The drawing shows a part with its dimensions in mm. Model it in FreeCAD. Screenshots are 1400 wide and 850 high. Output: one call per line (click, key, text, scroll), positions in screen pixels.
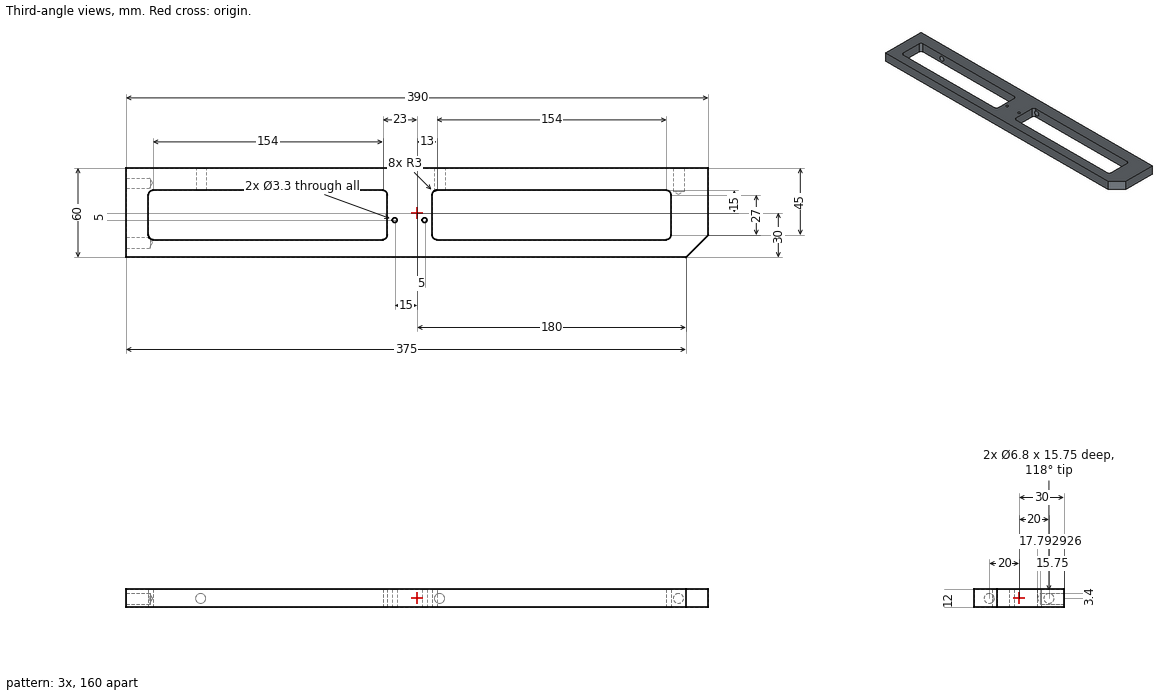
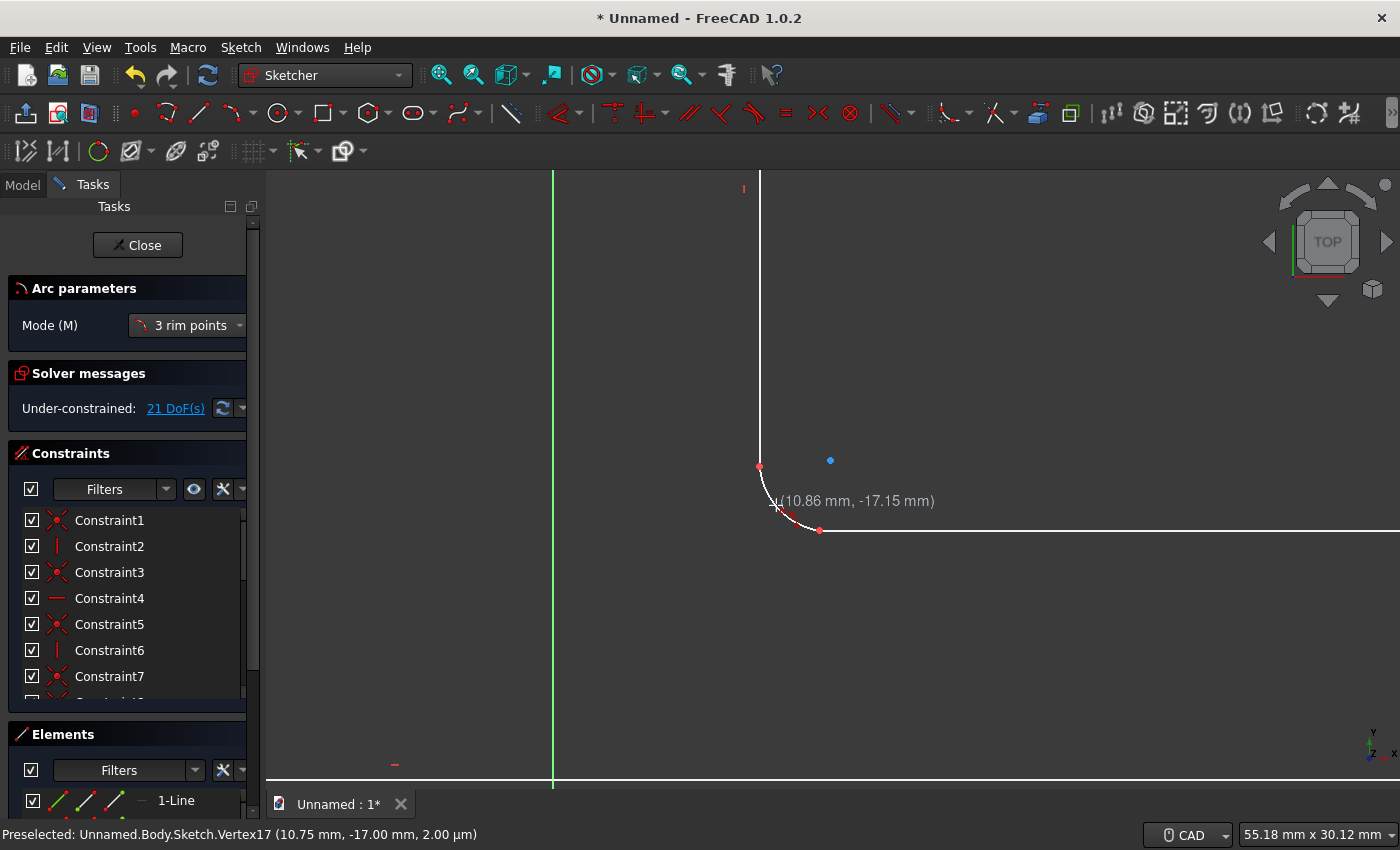
scroll(786, 512, down, 12)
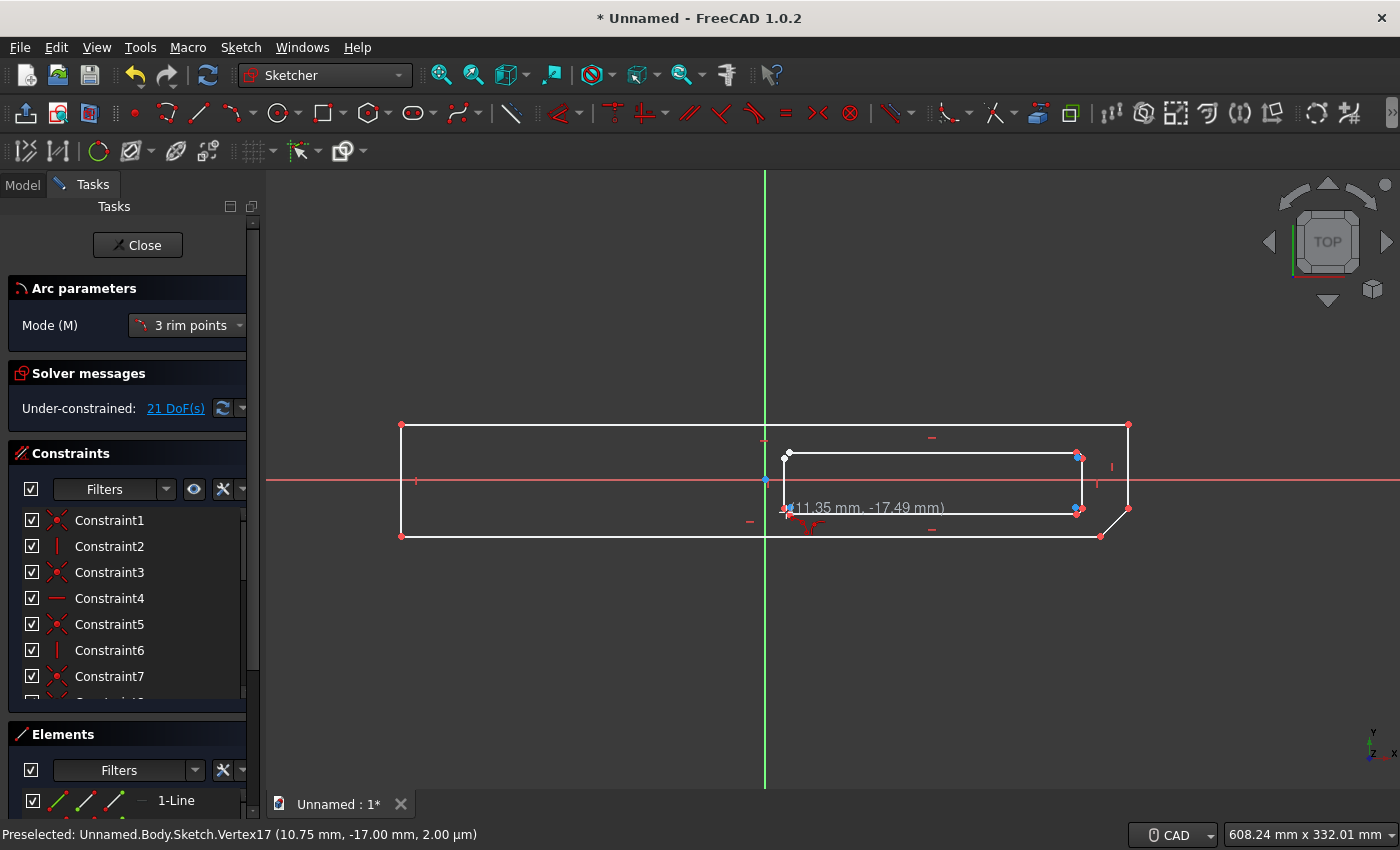
scroll(784, 458, up, 4)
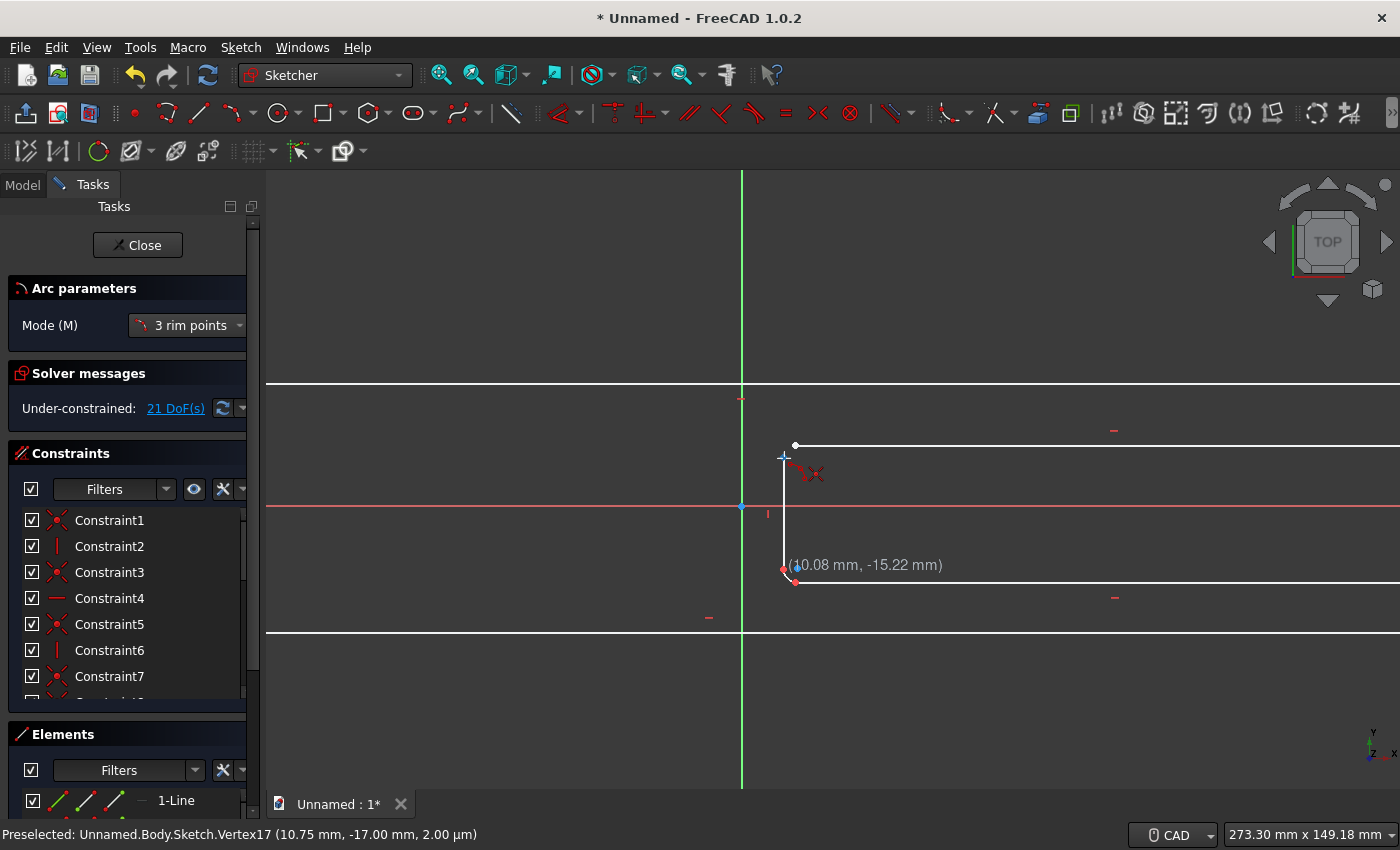
click(784, 458)
click(796, 446)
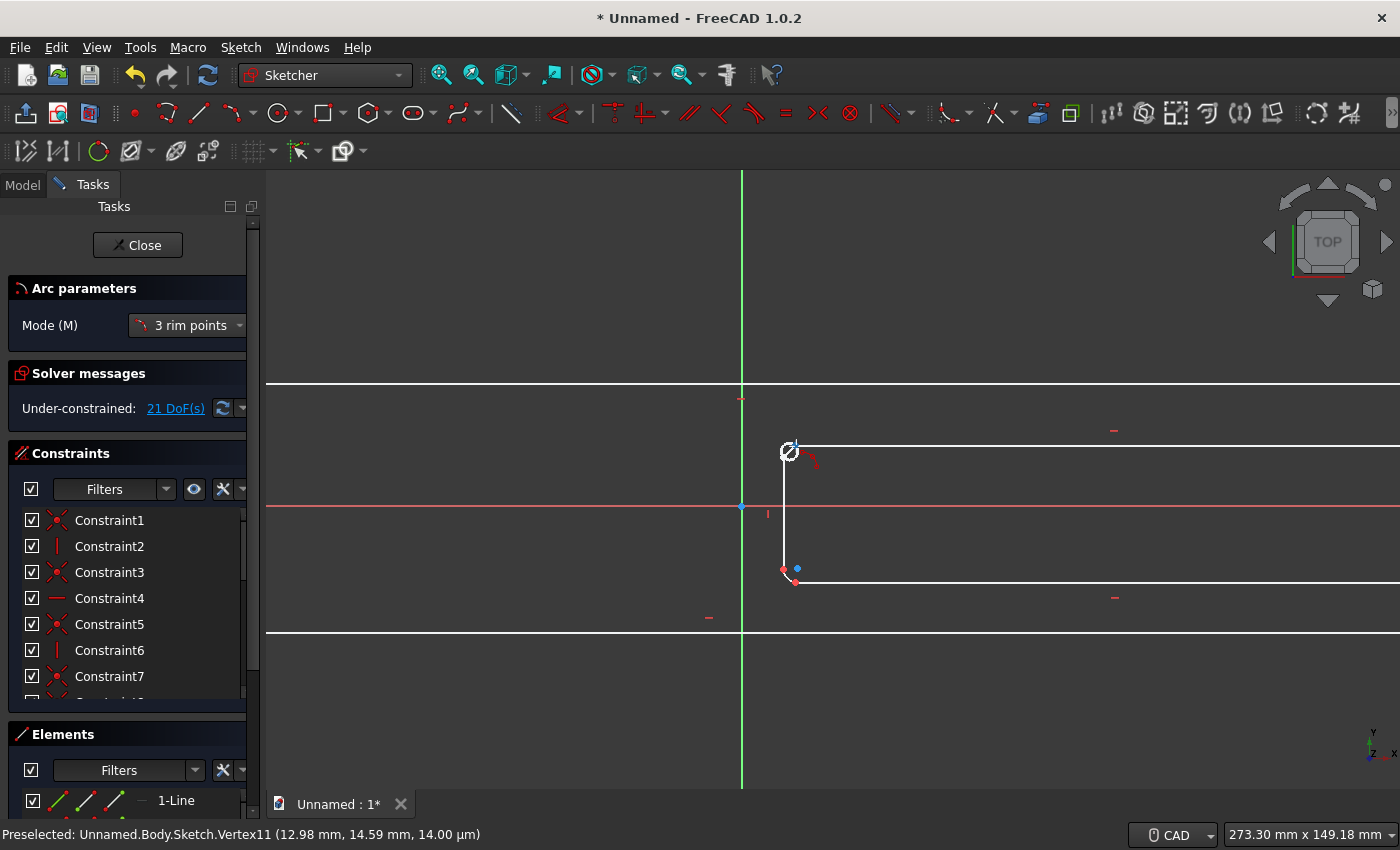
scroll(787, 448, up, 8)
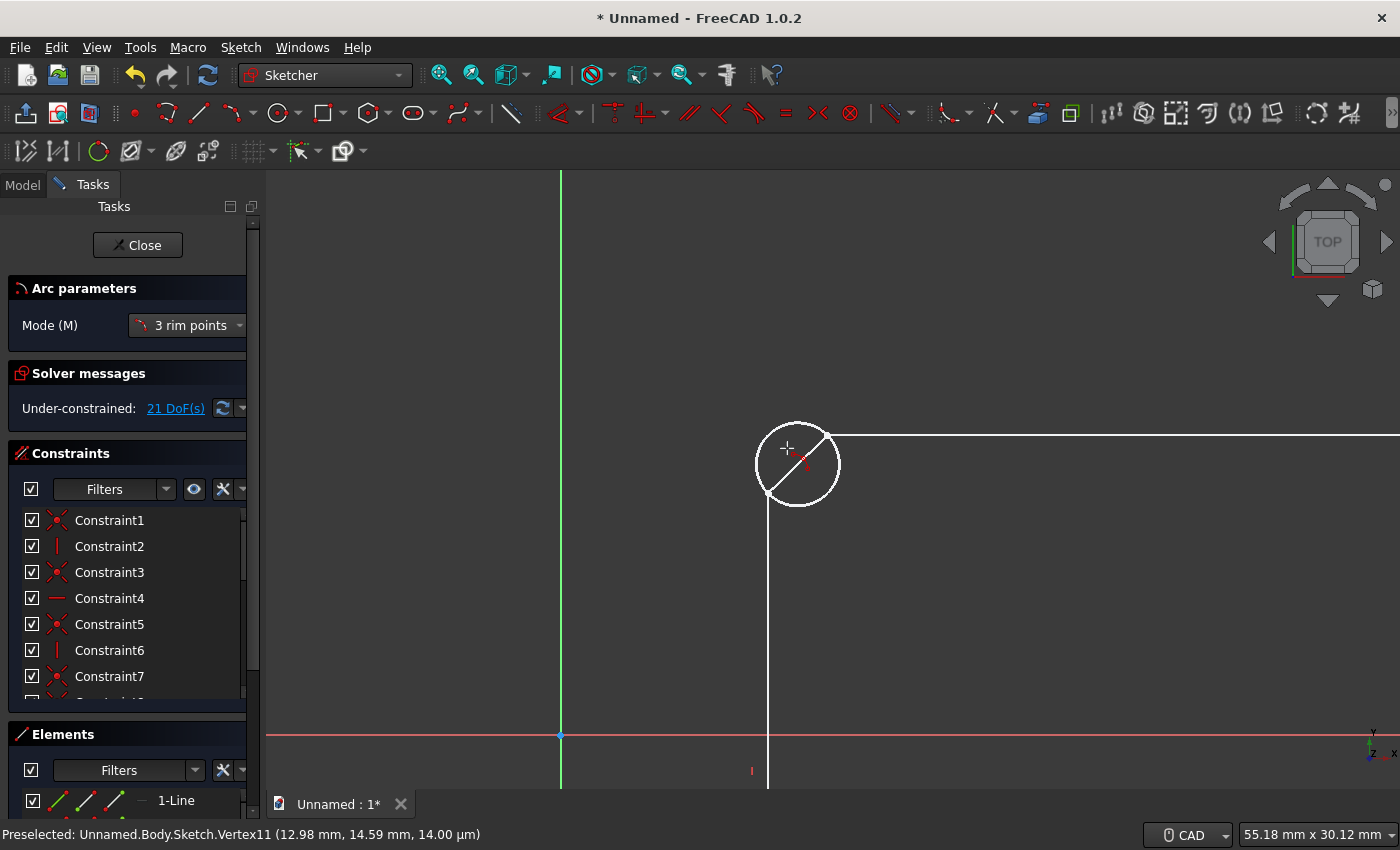
click(784, 445)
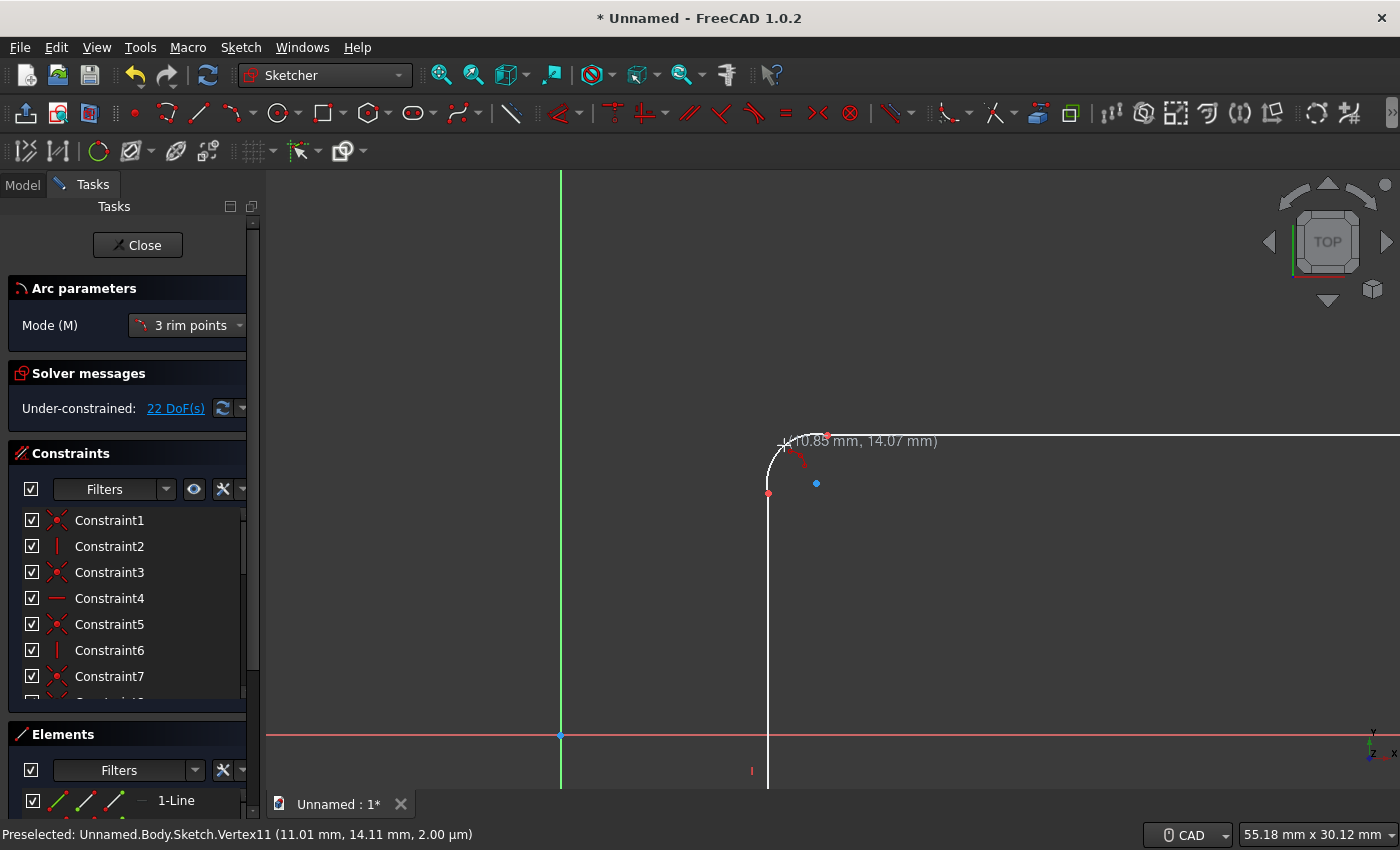
click(200, 114)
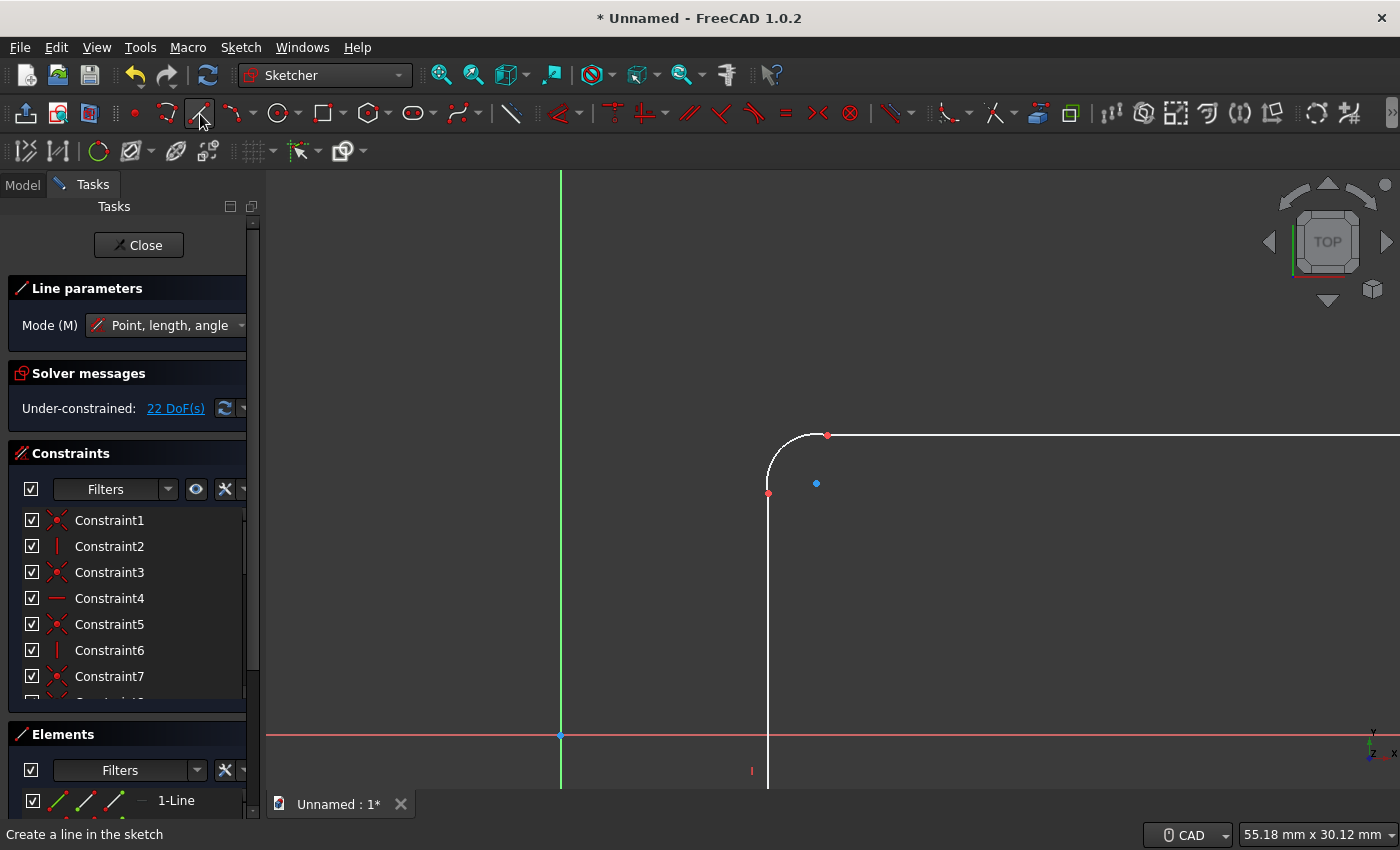
scroll(785, 454, down, 12)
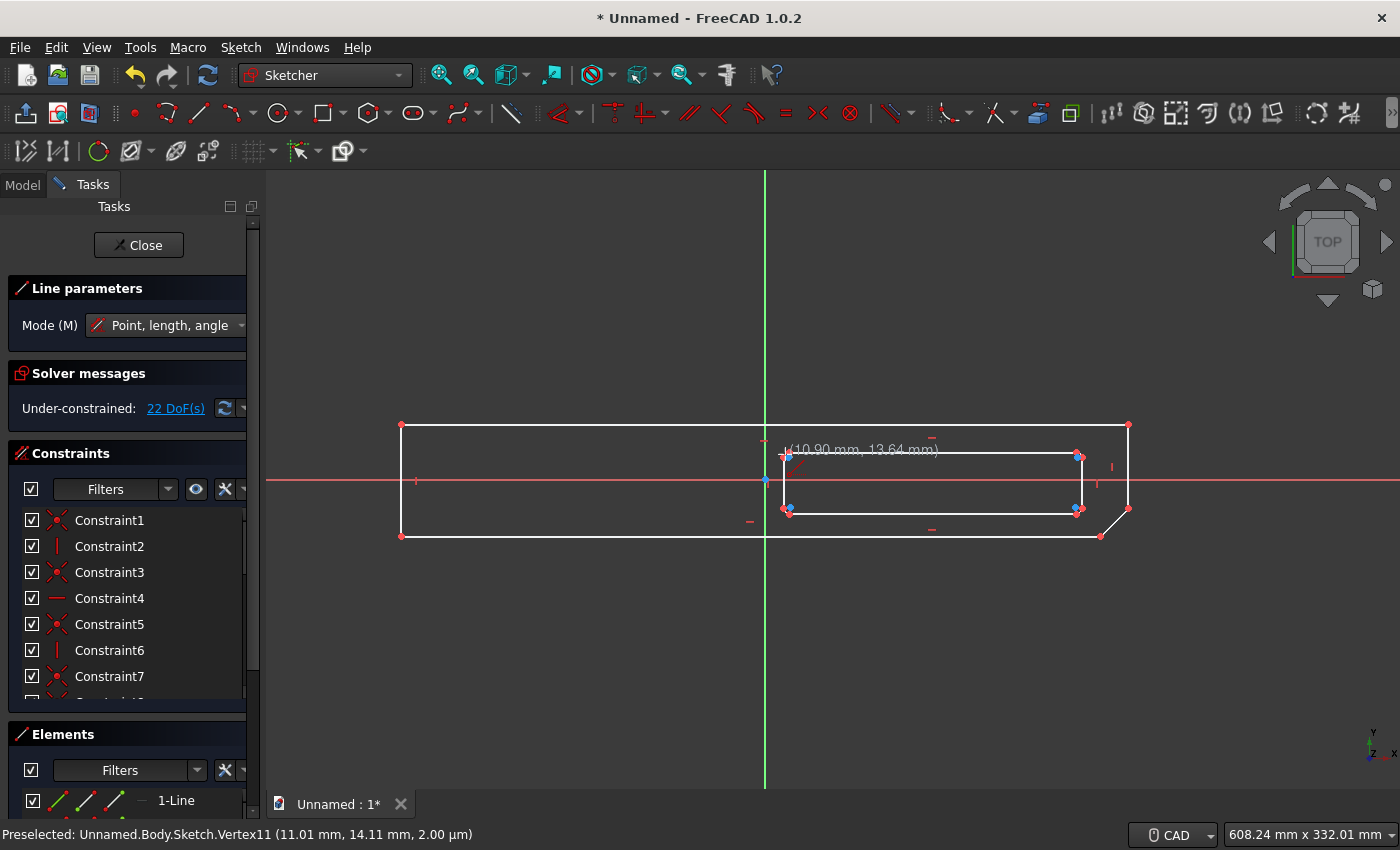
click(435, 452)
click(722, 452)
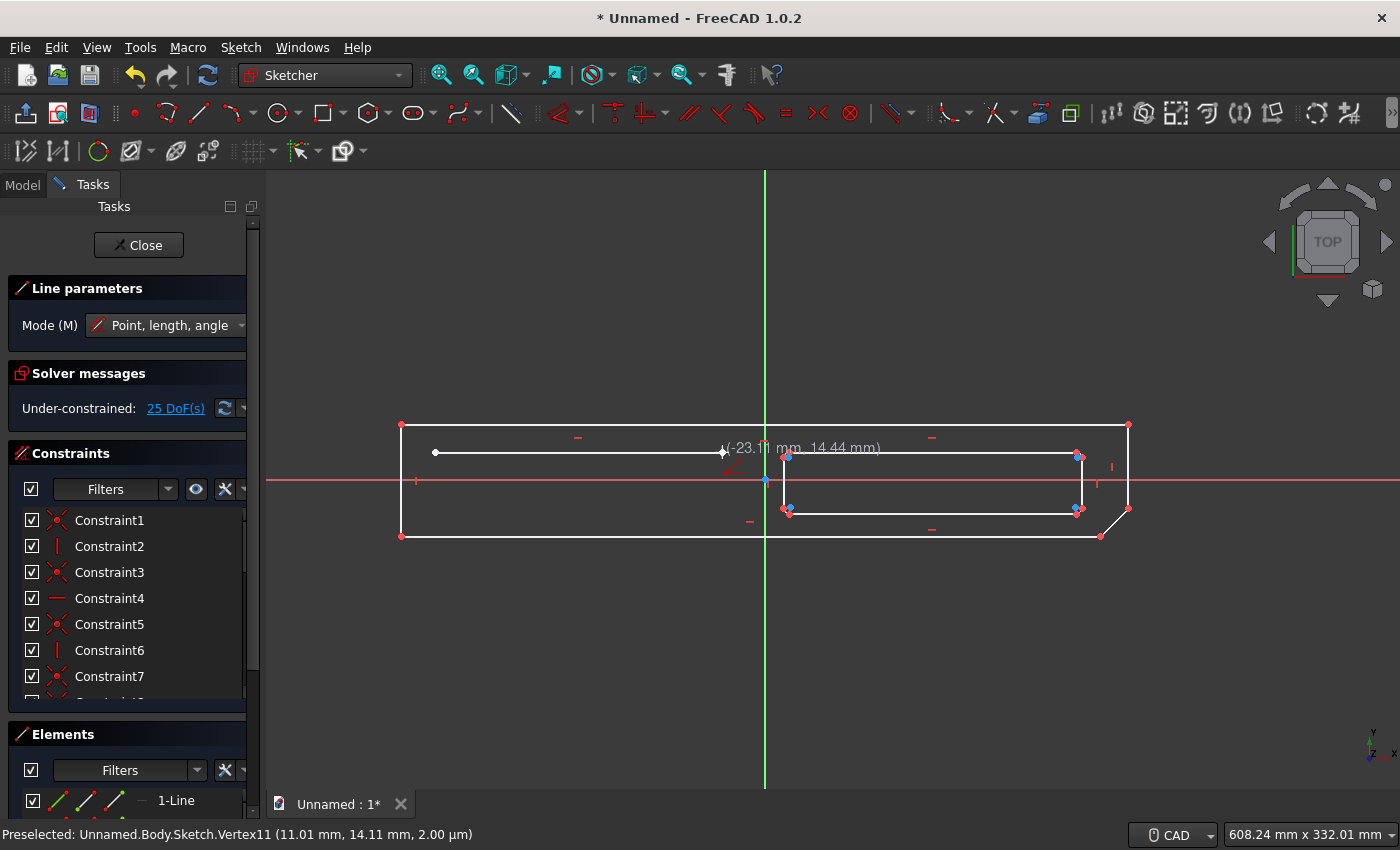
scroll(728, 458, up, 4)